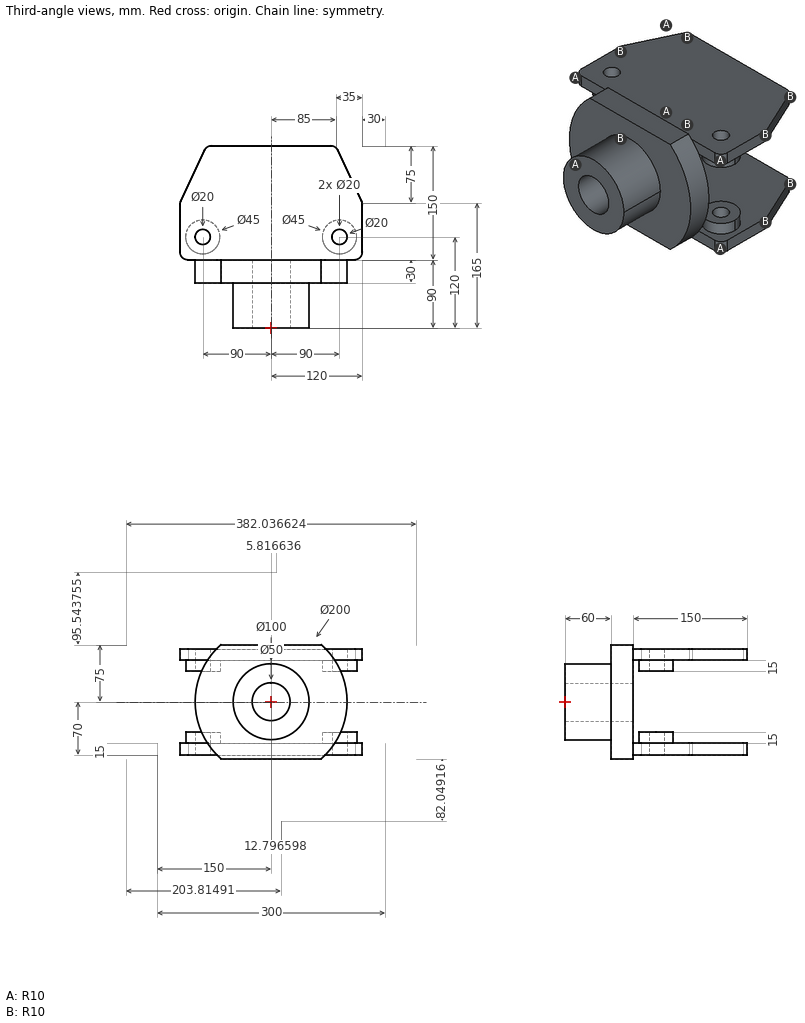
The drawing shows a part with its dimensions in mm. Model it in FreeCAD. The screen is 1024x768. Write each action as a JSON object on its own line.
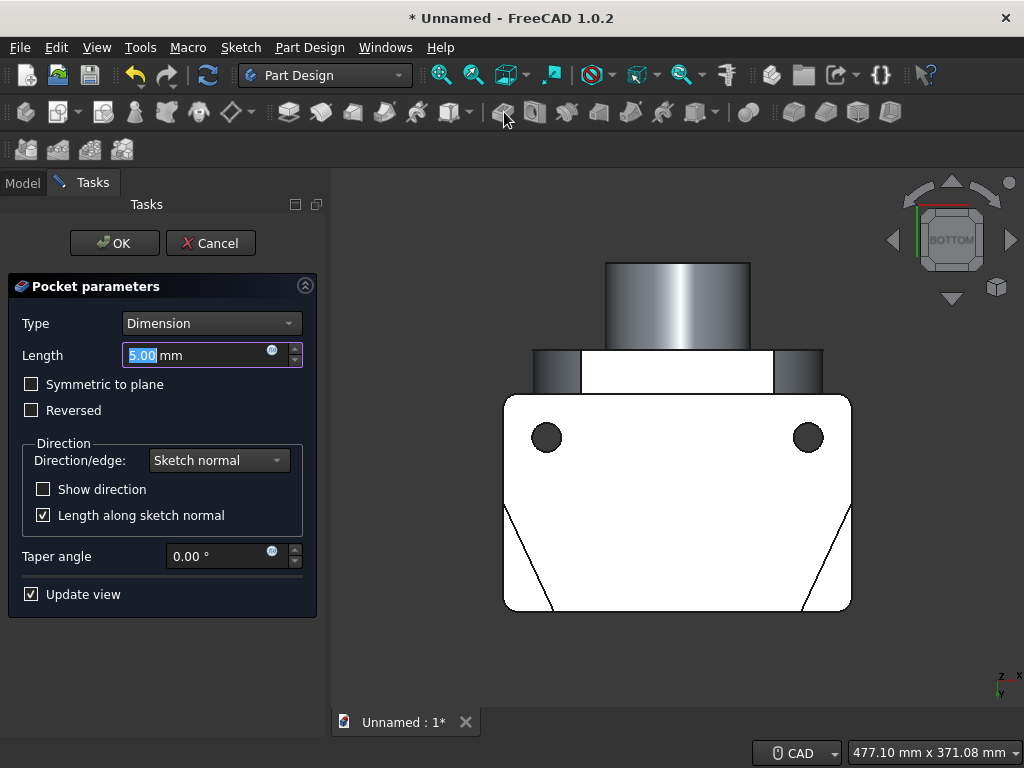
{"action": "left_click", "coordinate": [212, 324]}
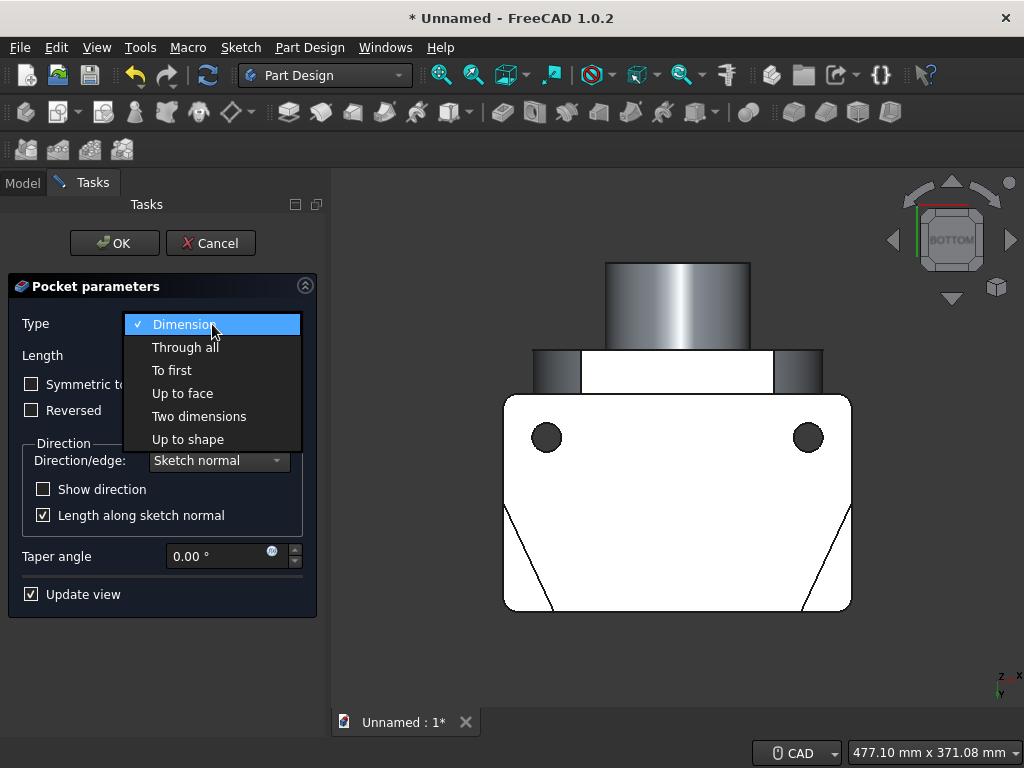
{"action": "left_click", "coordinate": [212, 348]}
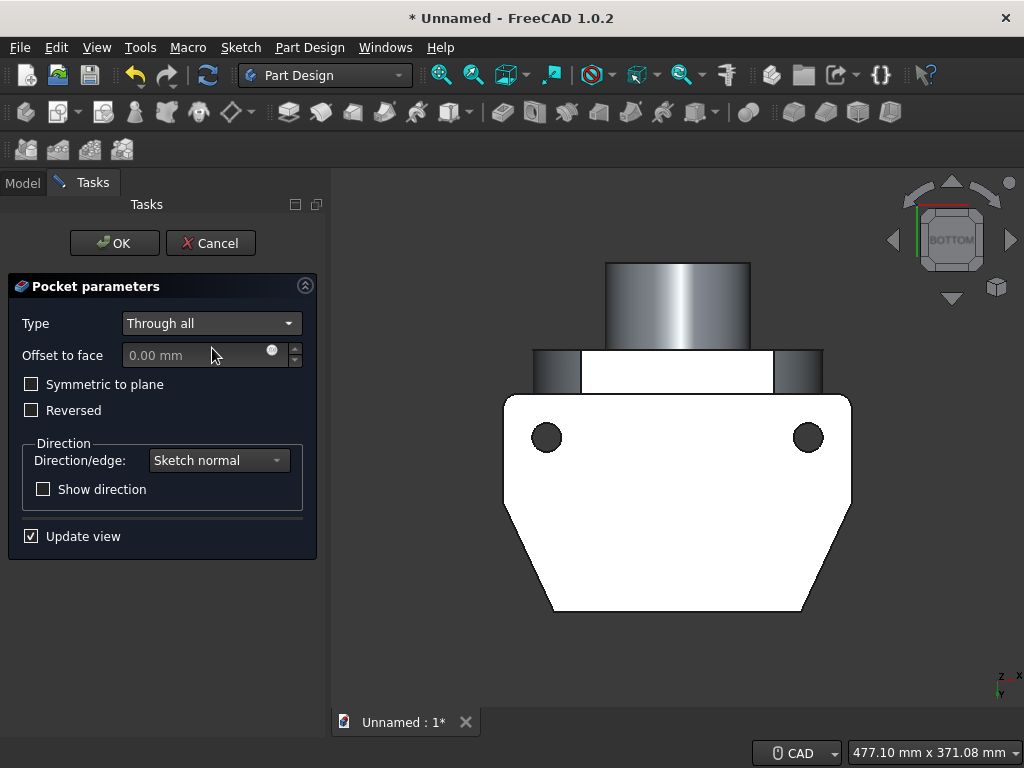
{"action": "left_click", "coordinate": [115, 243]}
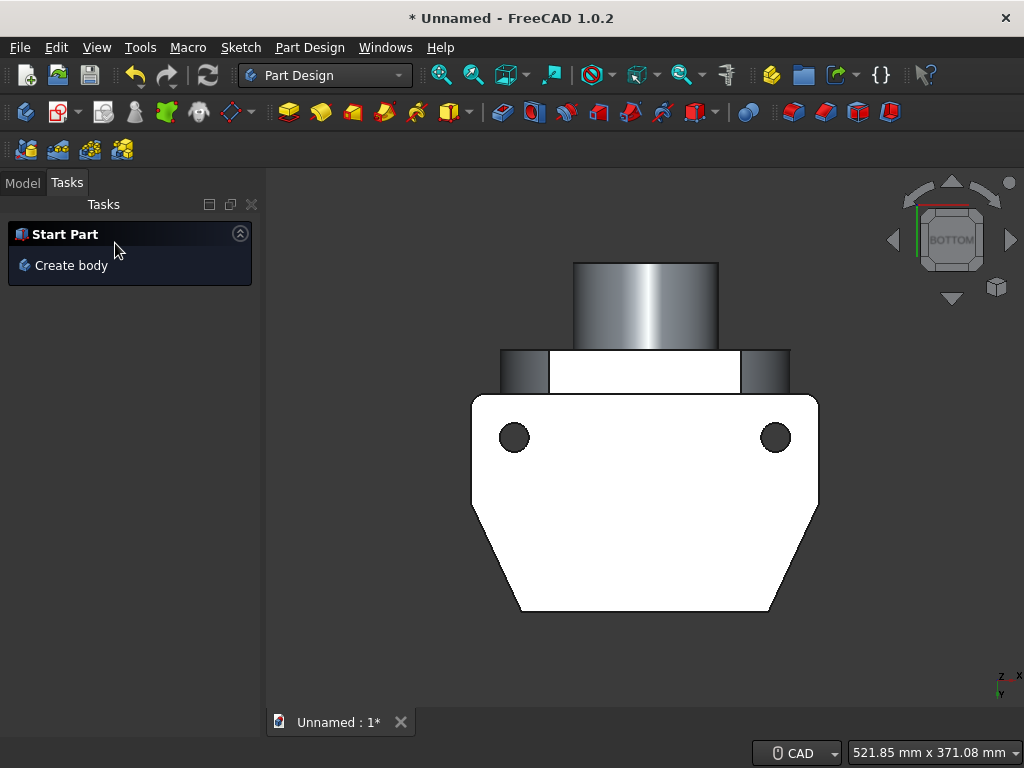
{"action": "scroll", "coordinate": [768, 611], "scroll_direction": "up", "scroll_amount": 4}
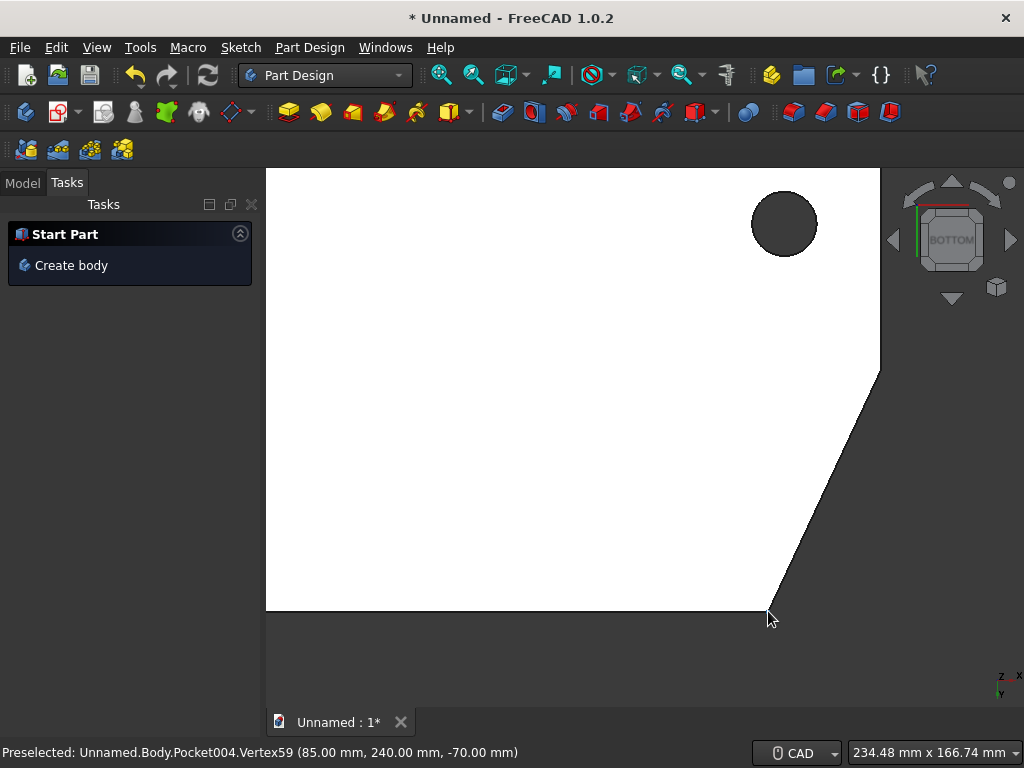
{"action": "left_click", "coordinate": [442, 76]}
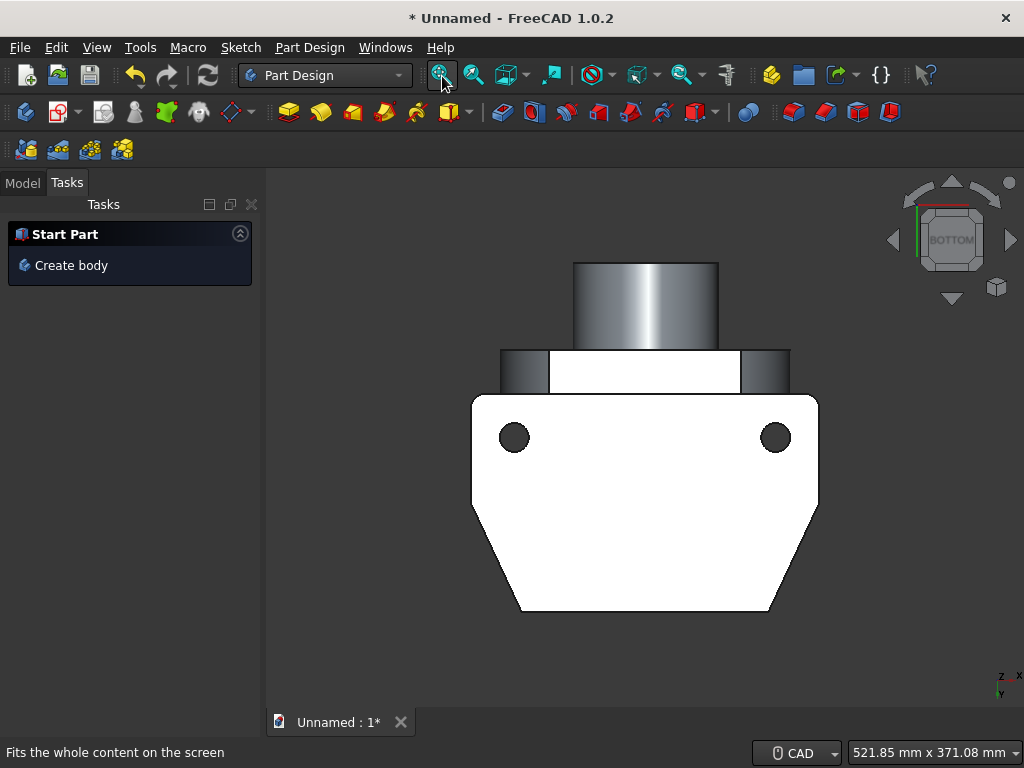
{"action": "key", "text": "0"}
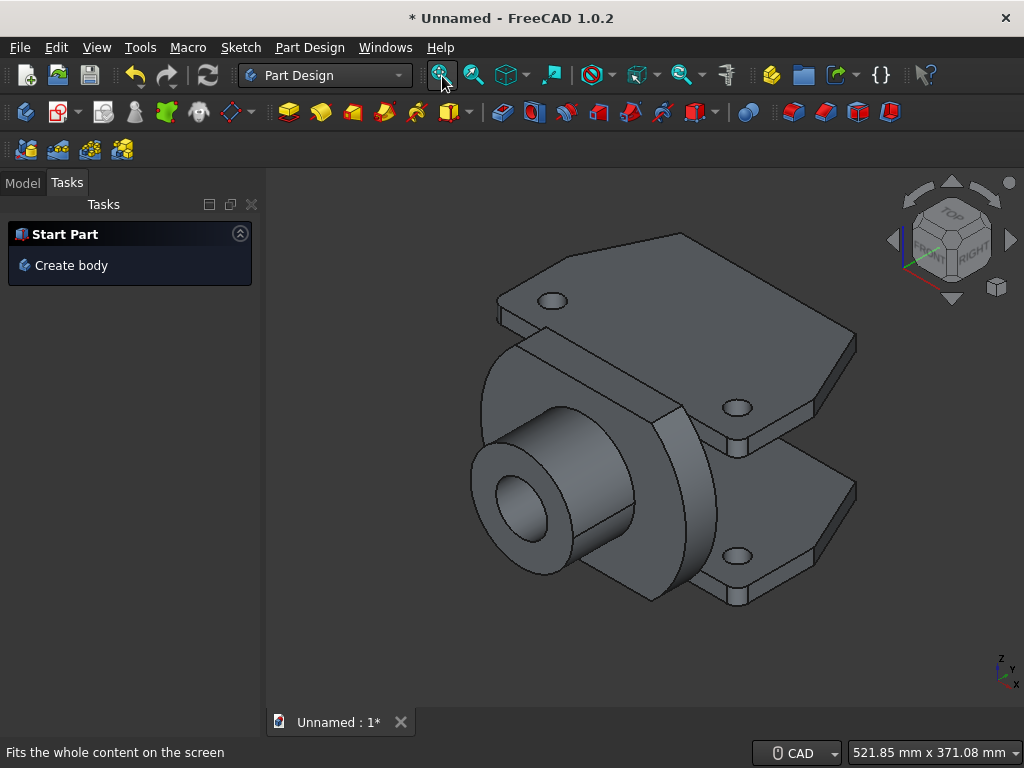
{"action": "scroll", "coordinate": [856, 490], "scroll_direction": "up", "scroll_amount": 4}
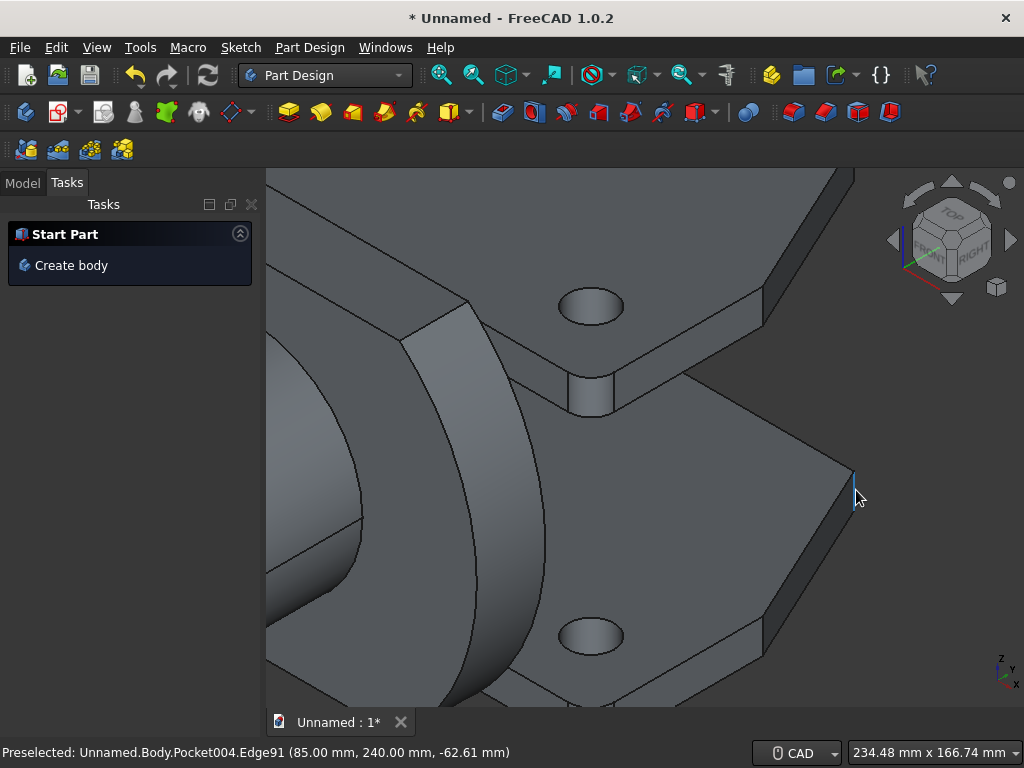
{"action": "left_click", "coordinate": [442, 76]}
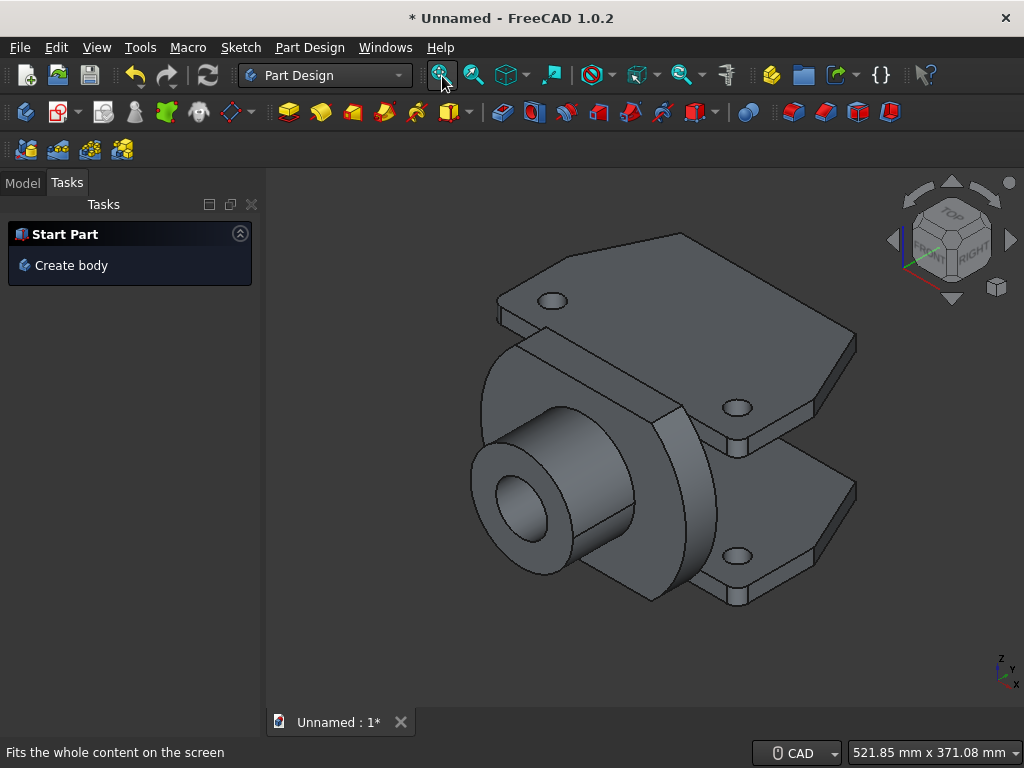
{"action": "key", "text": "2"}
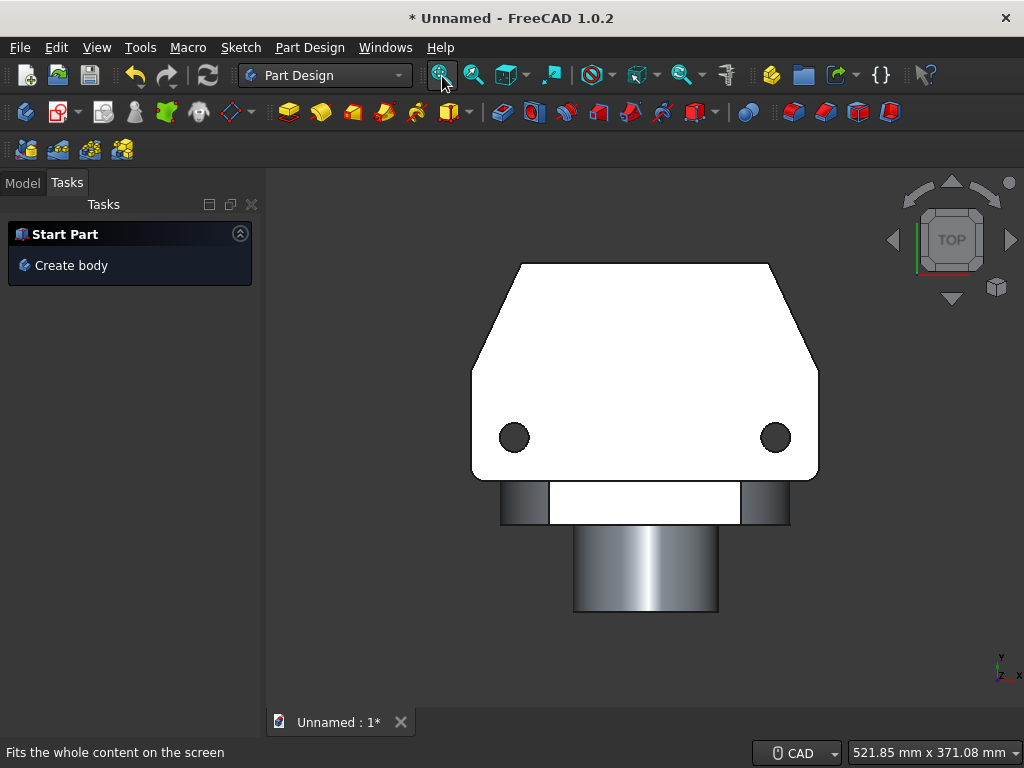
{"action": "scroll", "coordinate": [768, 262], "scroll_direction": "up", "scroll_amount": 4}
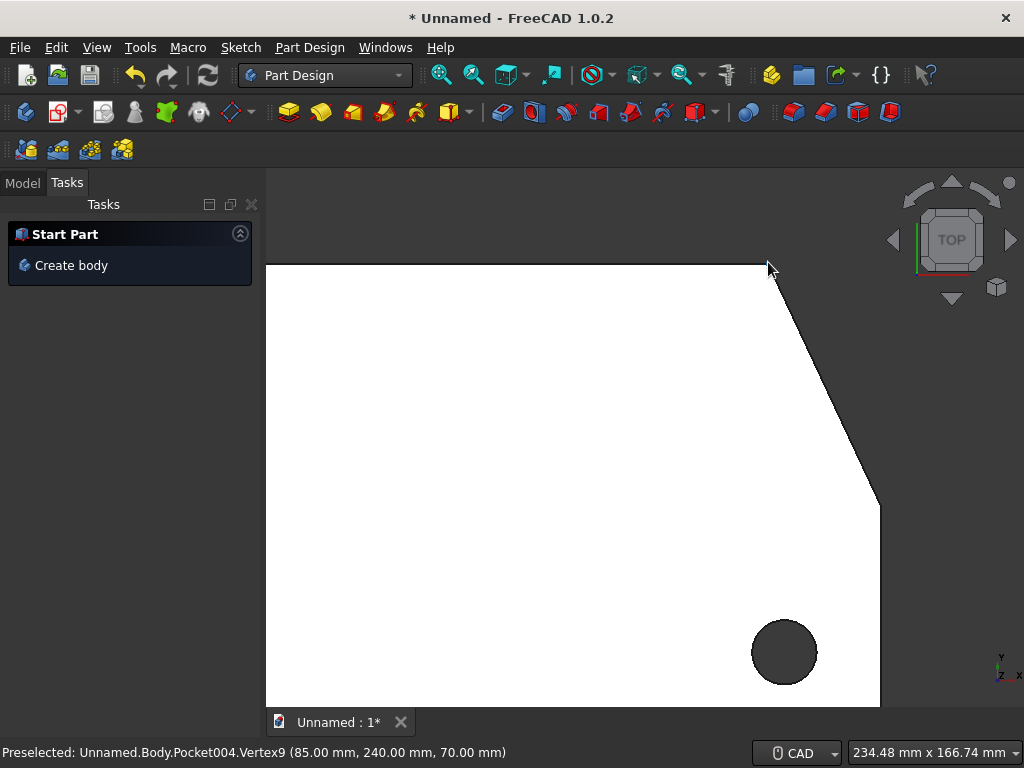
{"action": "left_click", "coordinate": [442, 76]}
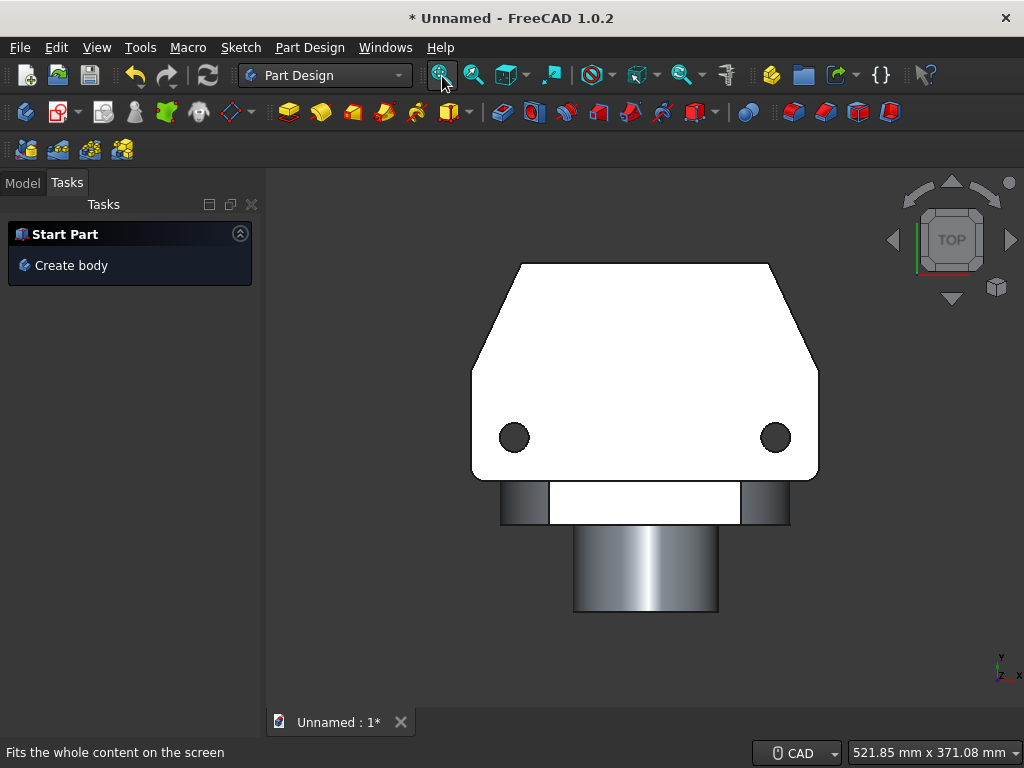
{"action": "key", "text": "1"}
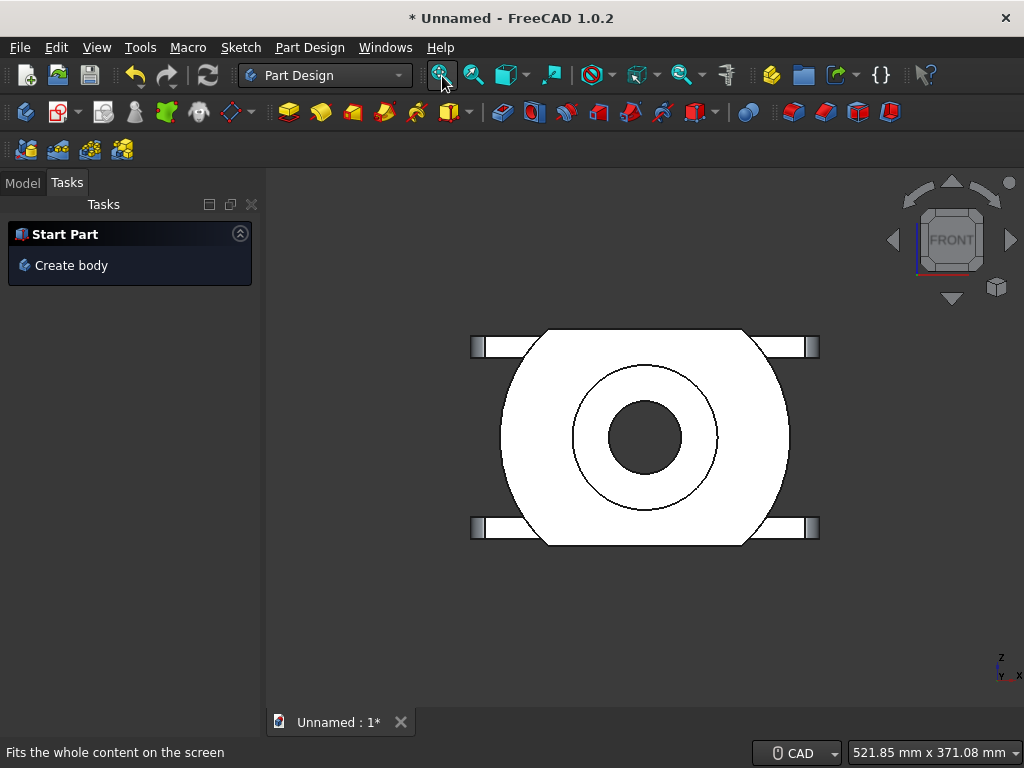
{"action": "scroll", "coordinate": [768, 527], "scroll_direction": "up", "scroll_amount": 4}